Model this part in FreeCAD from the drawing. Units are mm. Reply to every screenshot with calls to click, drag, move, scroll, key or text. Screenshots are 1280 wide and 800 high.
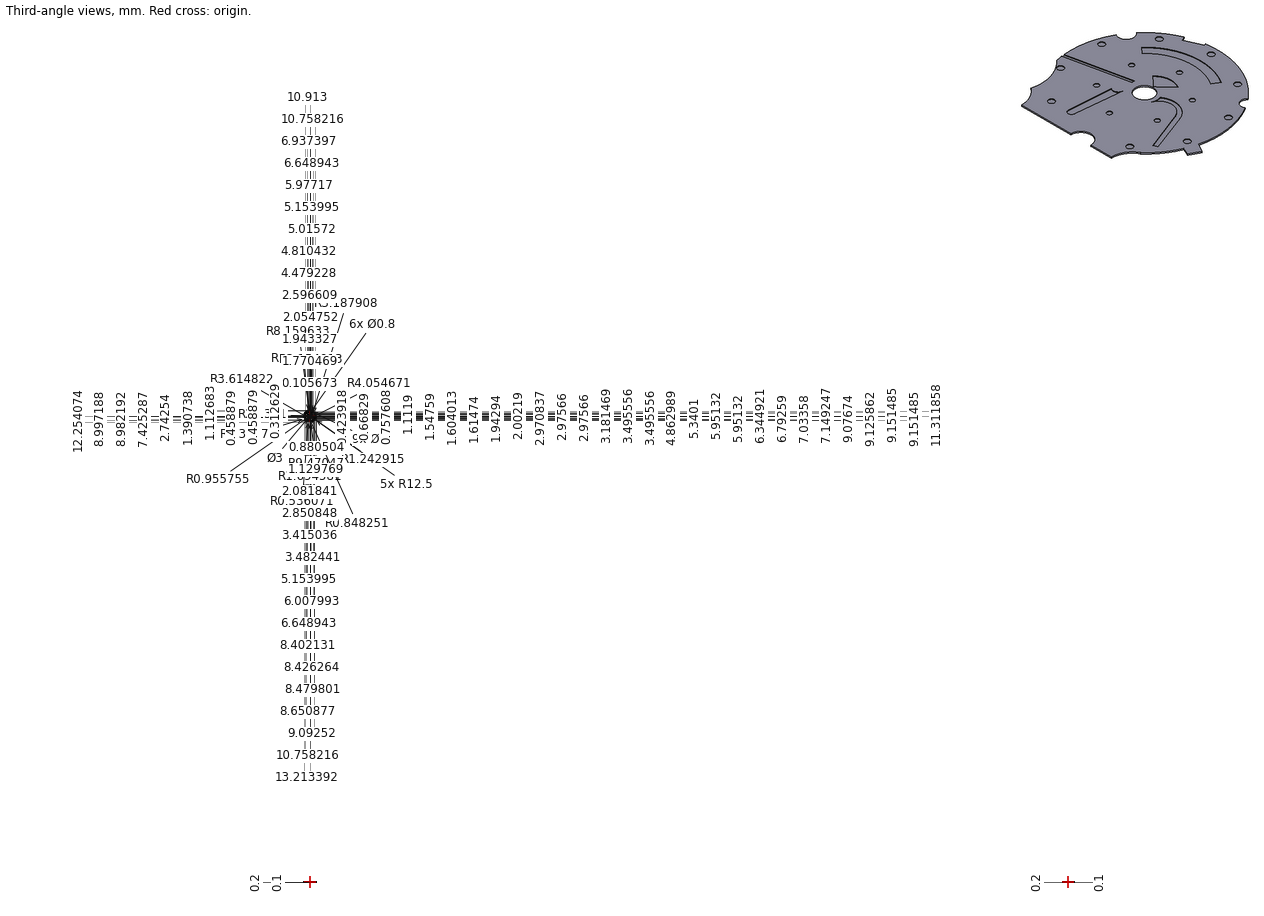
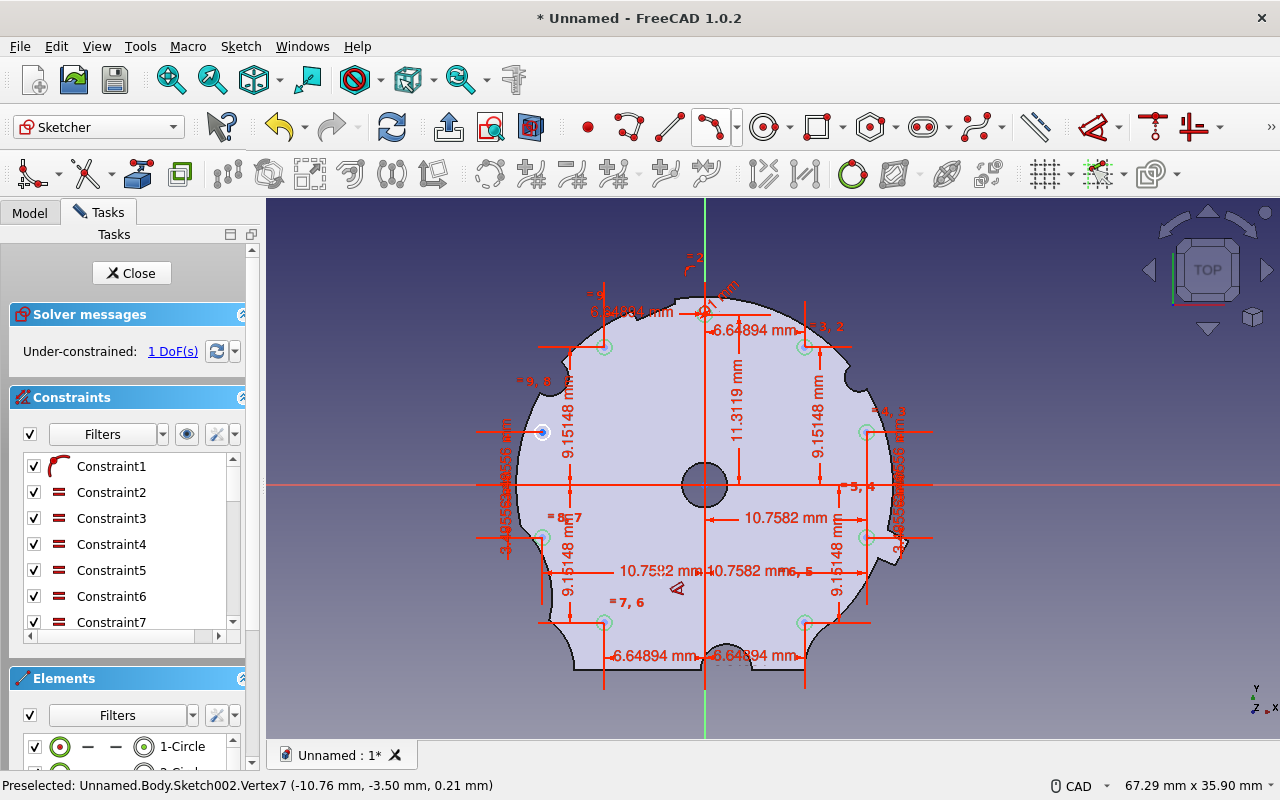
click(542, 432)
click(661, 398)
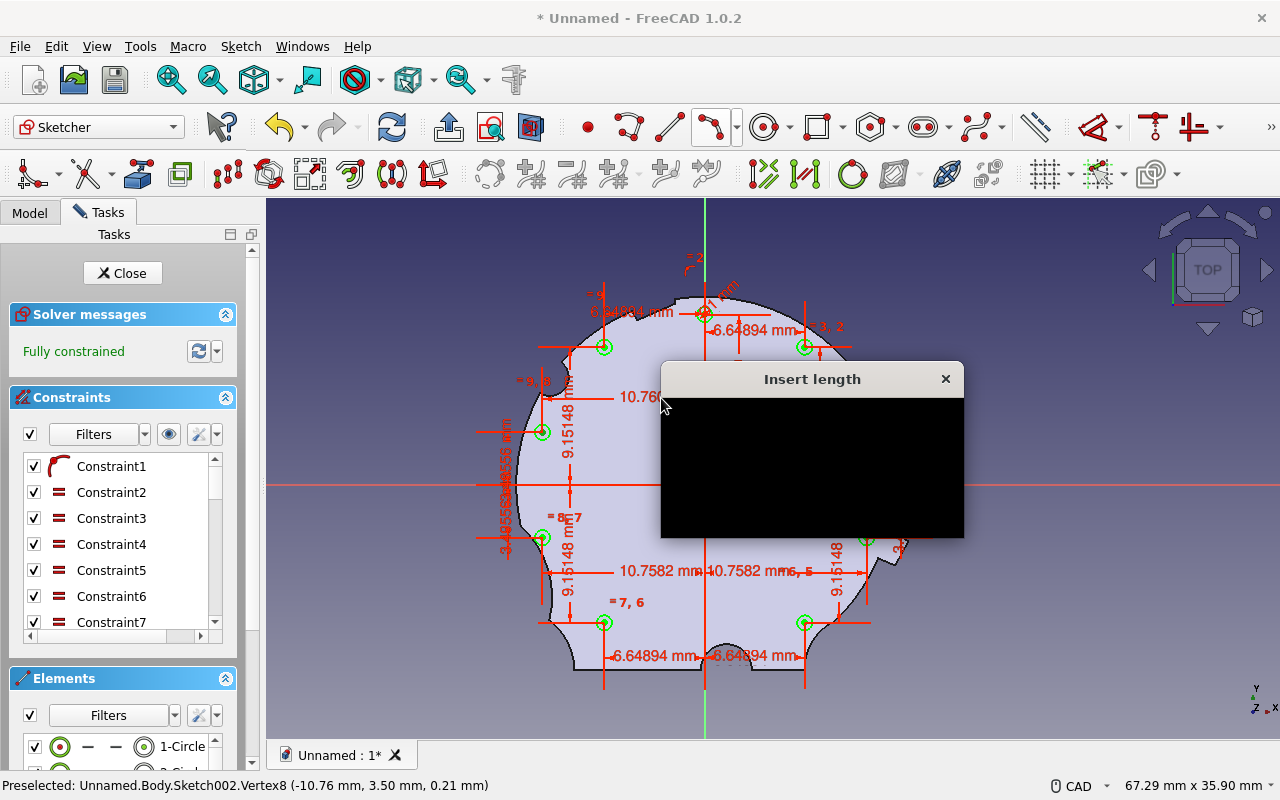
text(10.758216)
key(Return)
key(Escape)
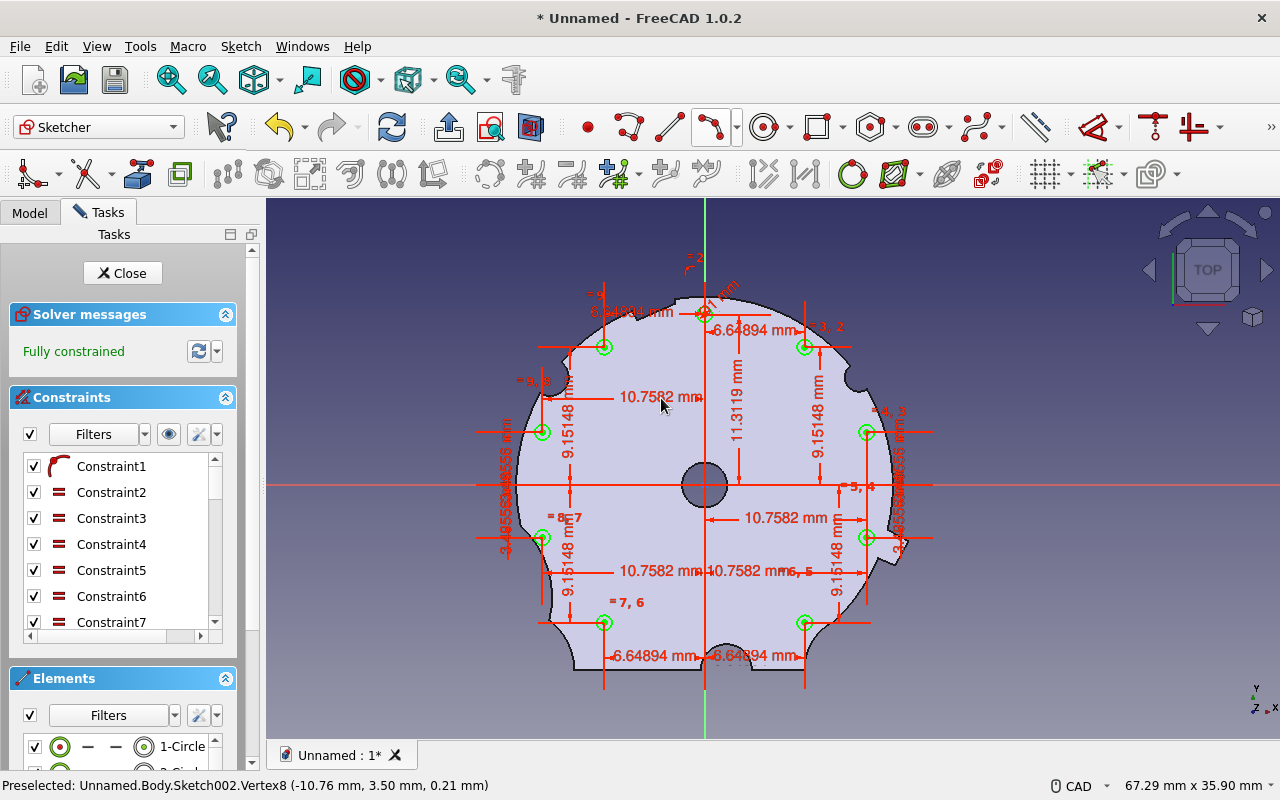
click(123, 273)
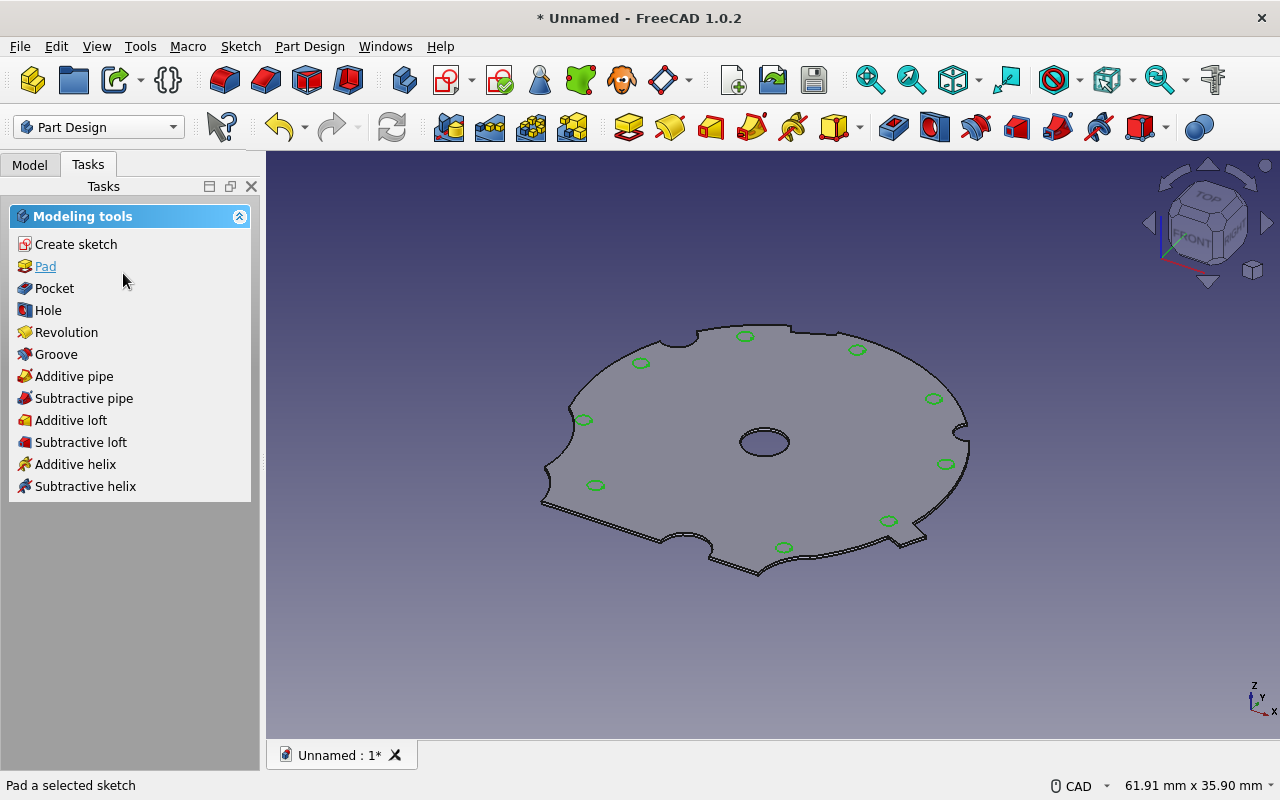
click(894, 128)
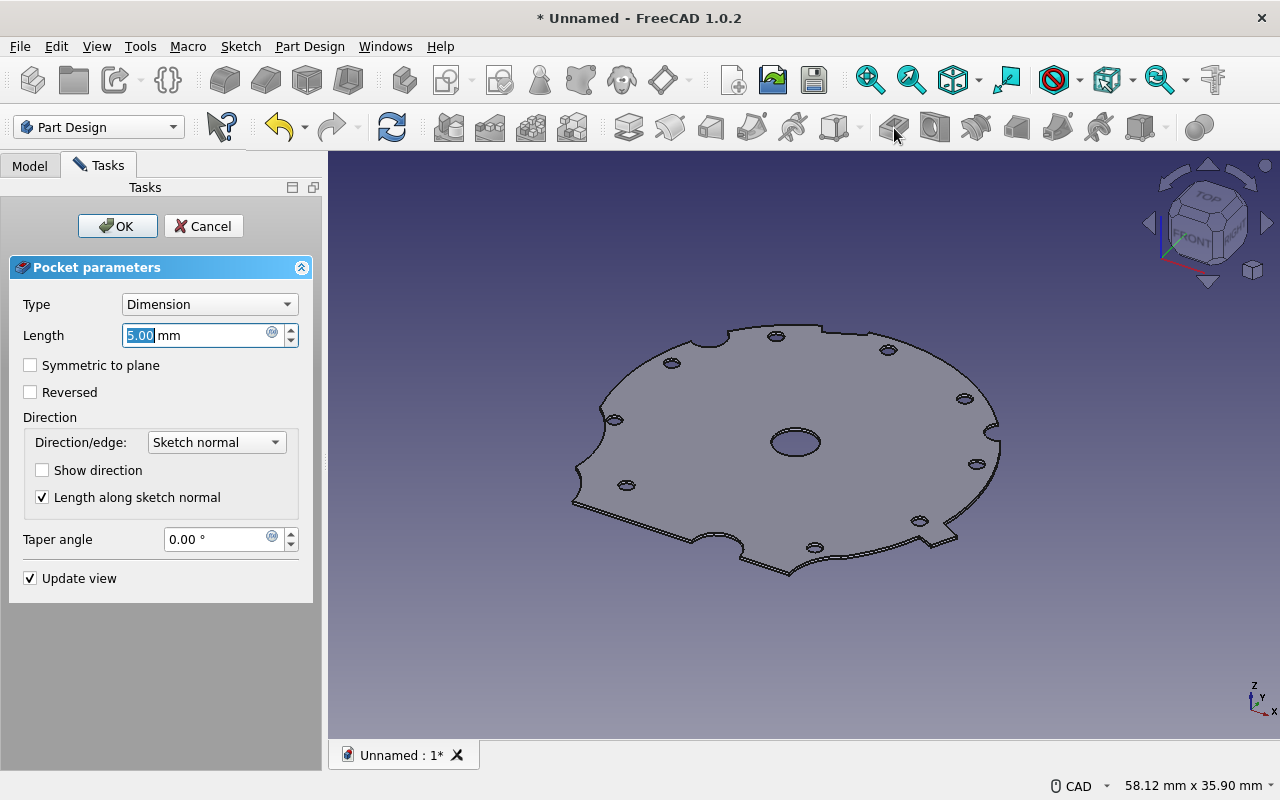
text(0.1)
key(Tab)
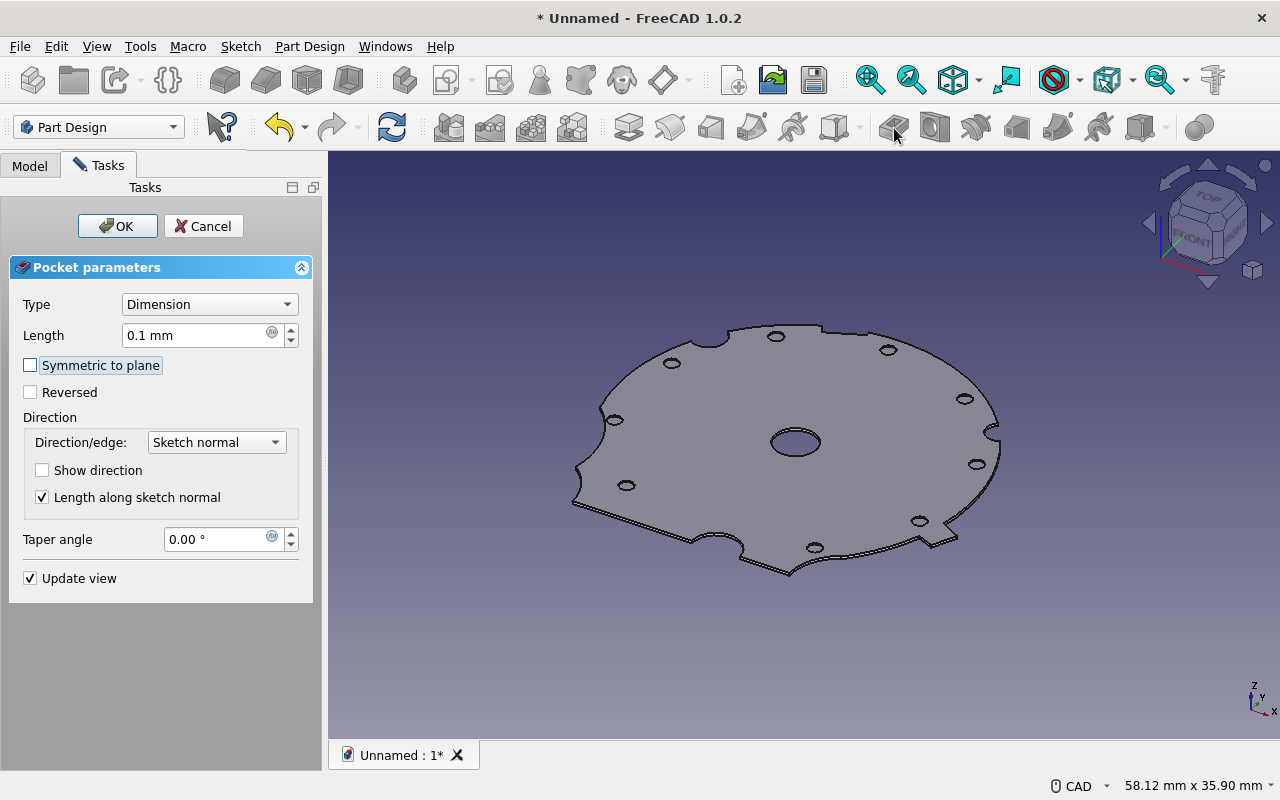
click(118, 226)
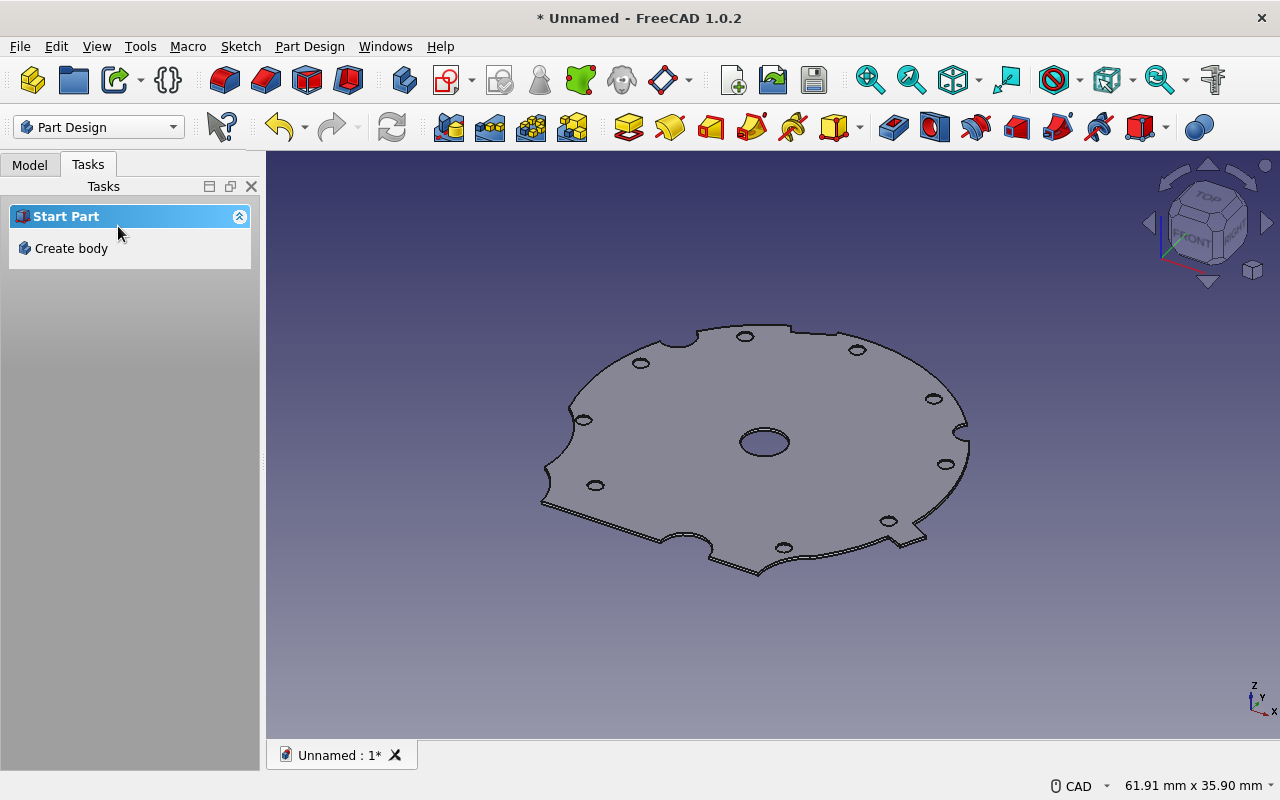
click(668, 408)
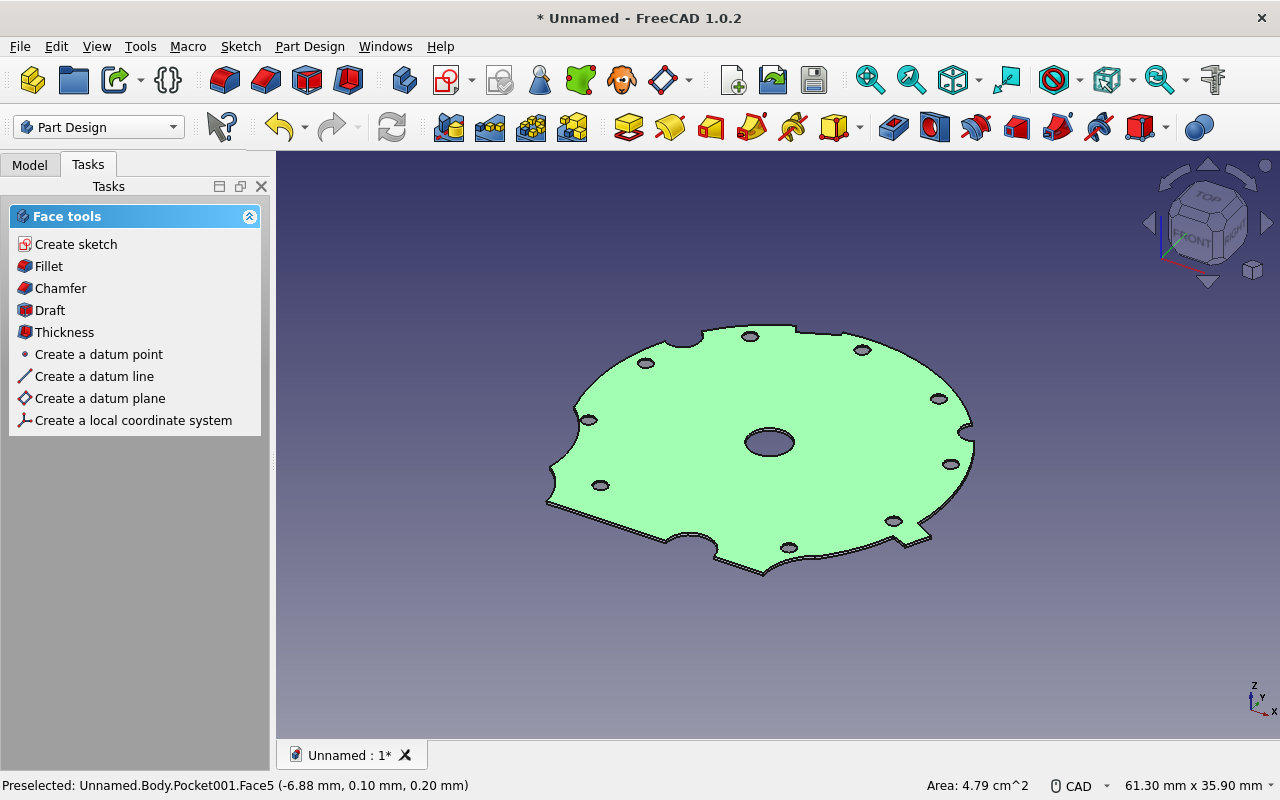
click(446, 80)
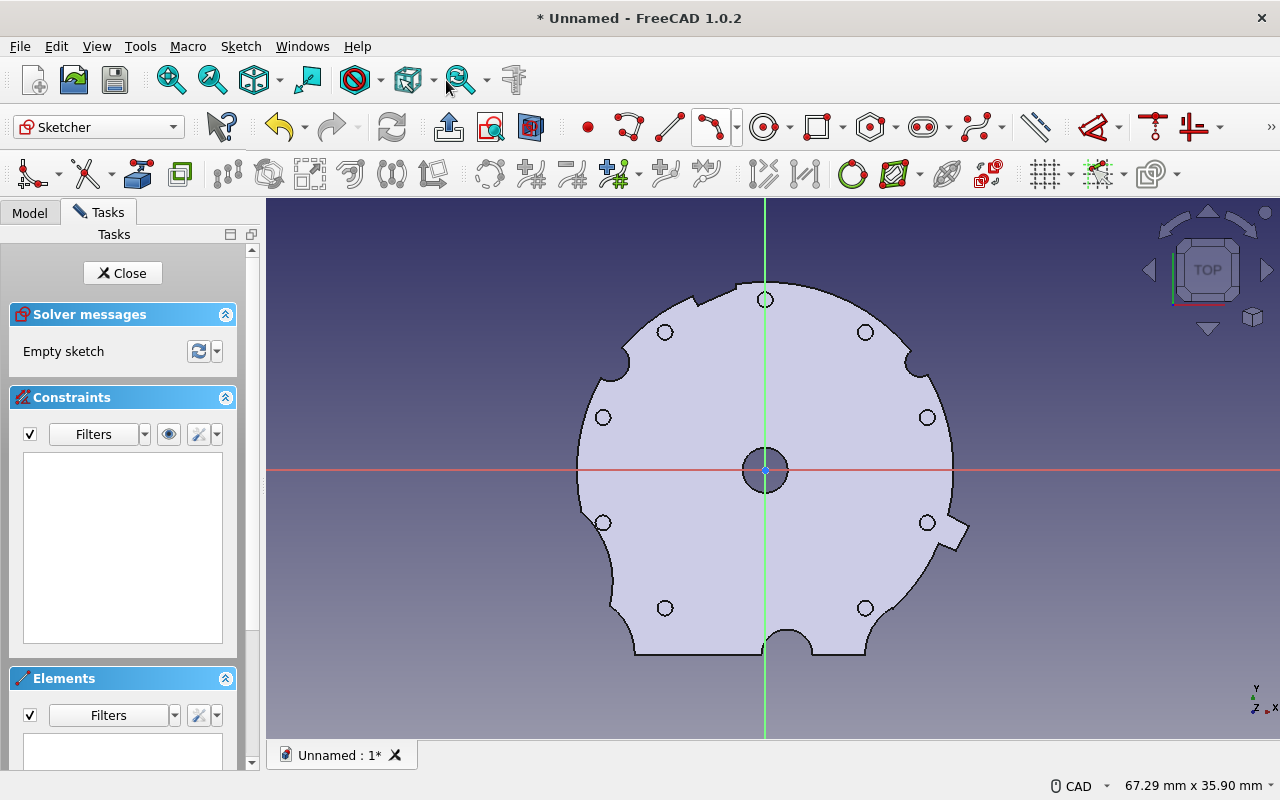
scroll(839, 472, up, 3)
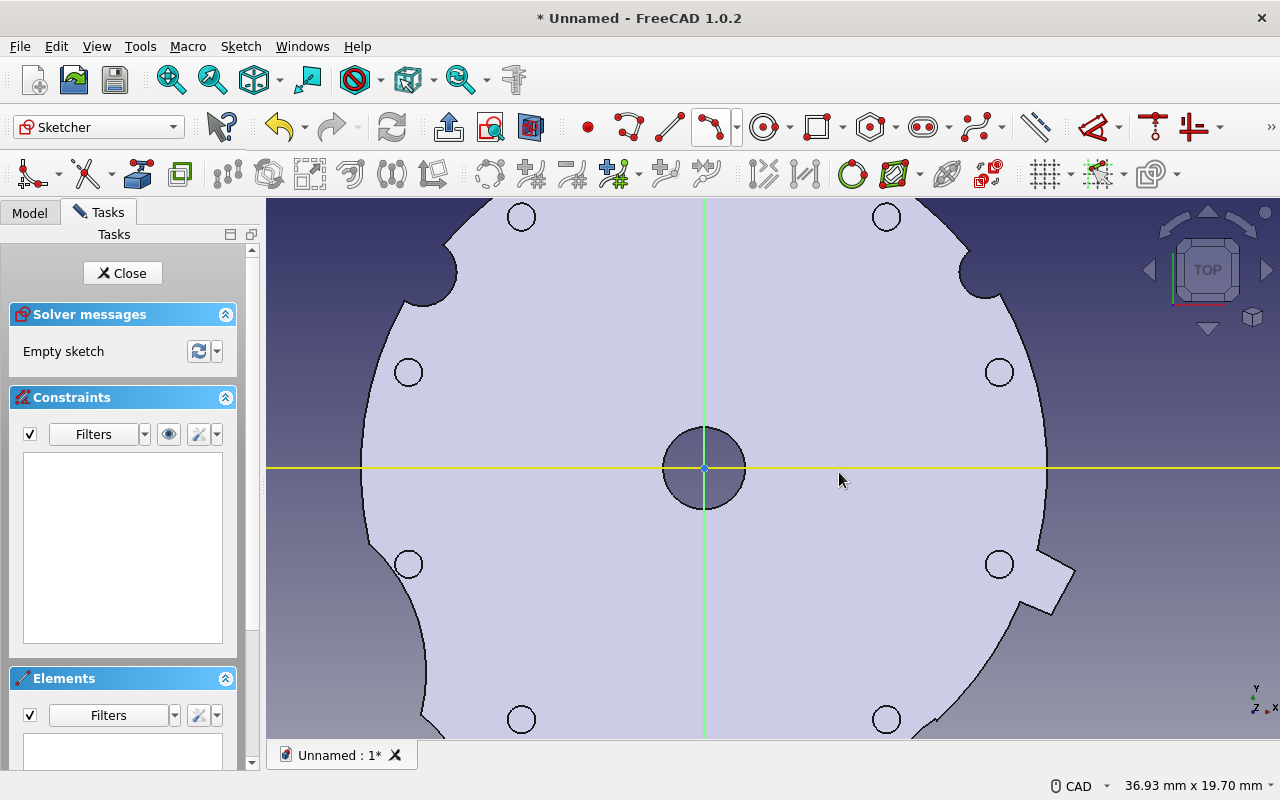
click(764, 128)